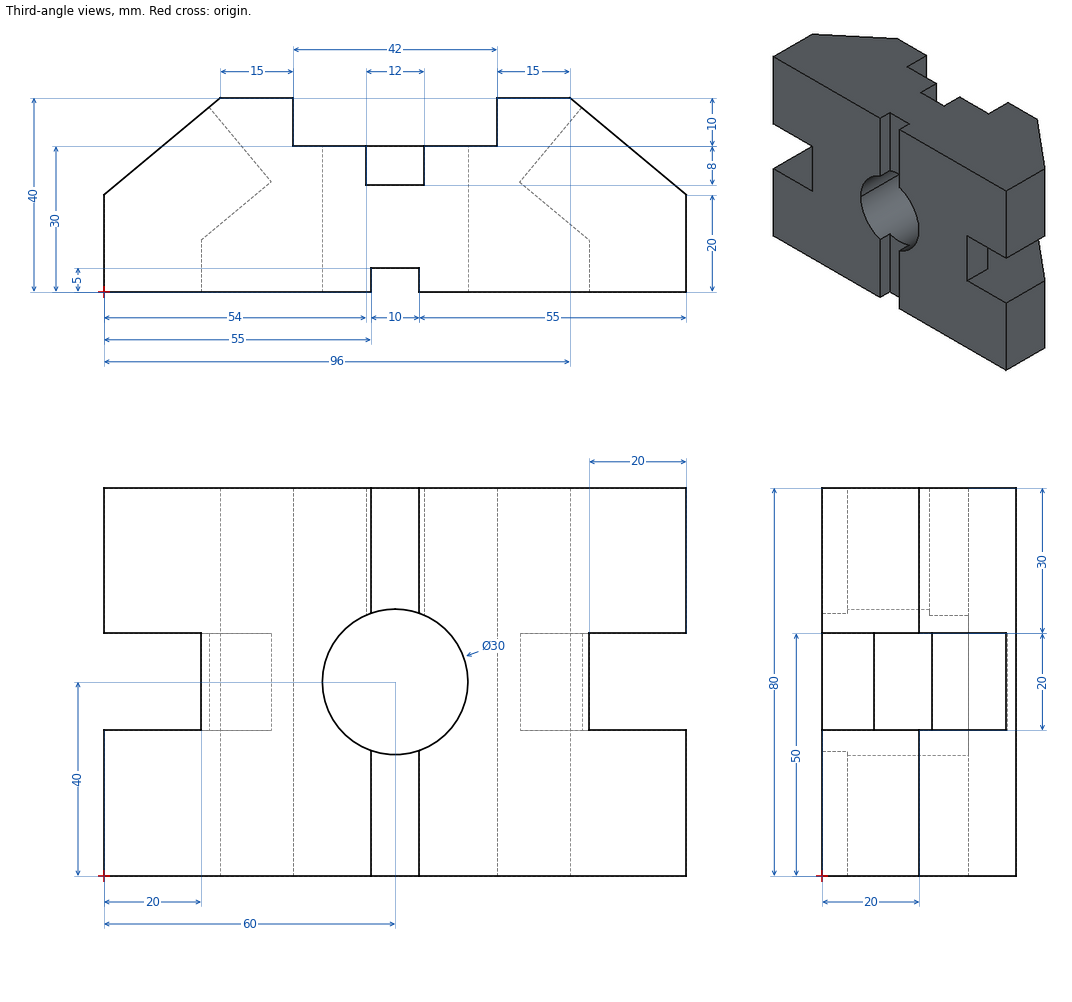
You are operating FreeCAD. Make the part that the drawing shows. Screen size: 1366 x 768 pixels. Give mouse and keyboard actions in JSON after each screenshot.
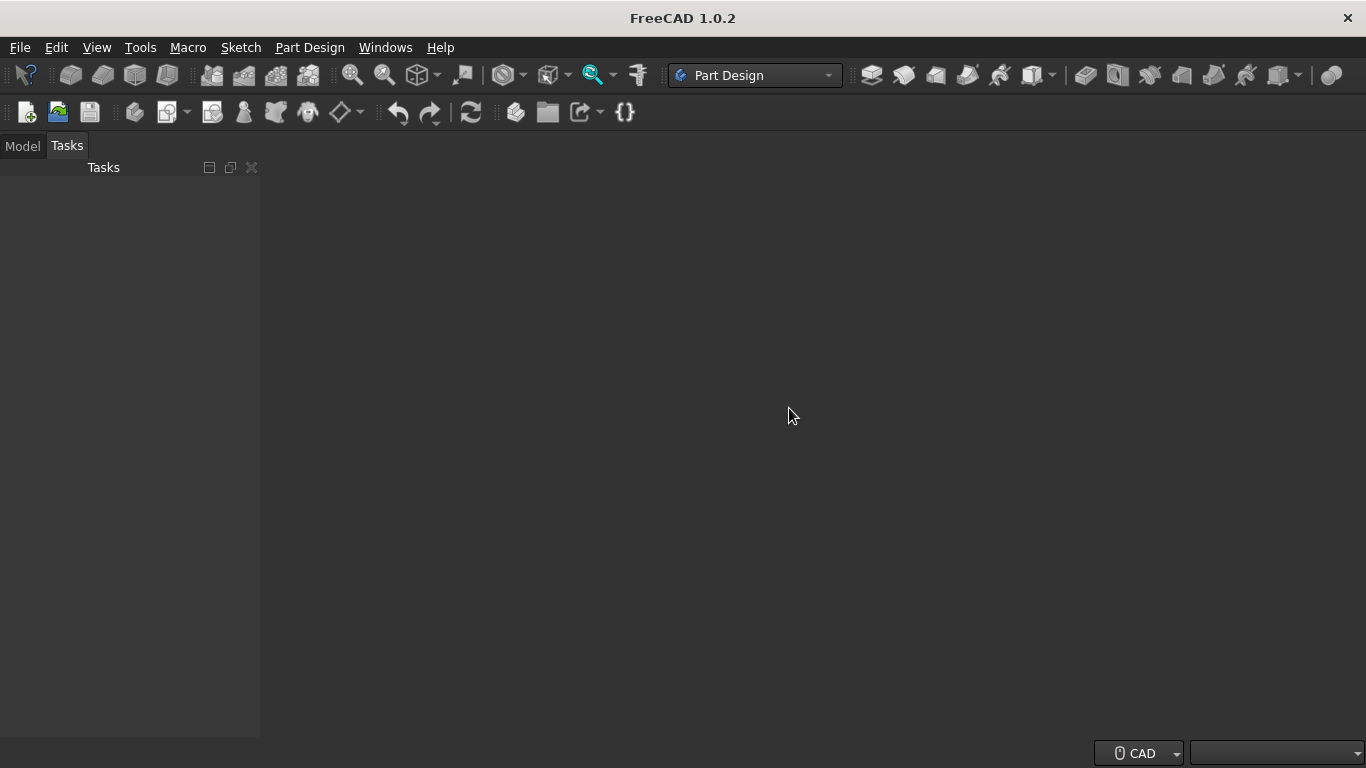
{"action": "left_click", "coordinate": [26, 112]}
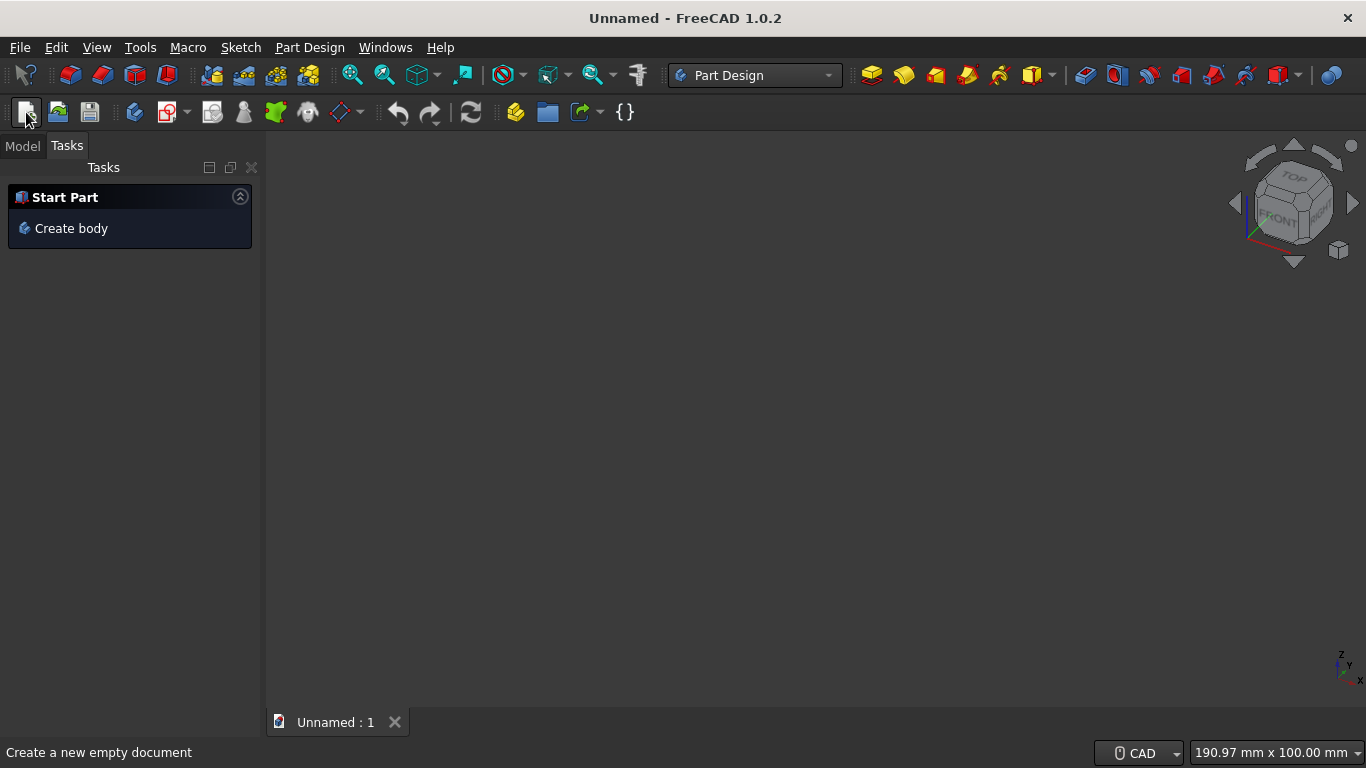
{"action": "left_click", "coordinate": [168, 112]}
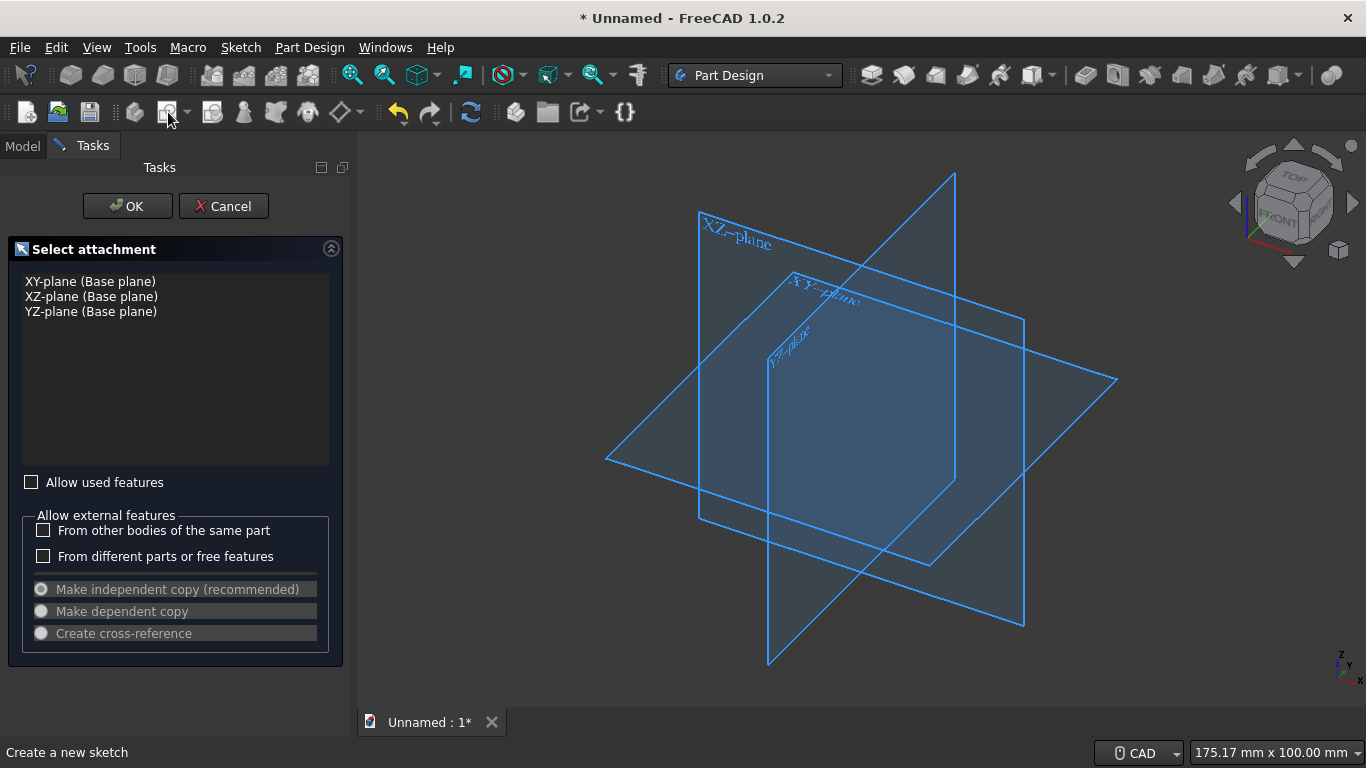
{"action": "left_click", "coordinate": [82, 282]}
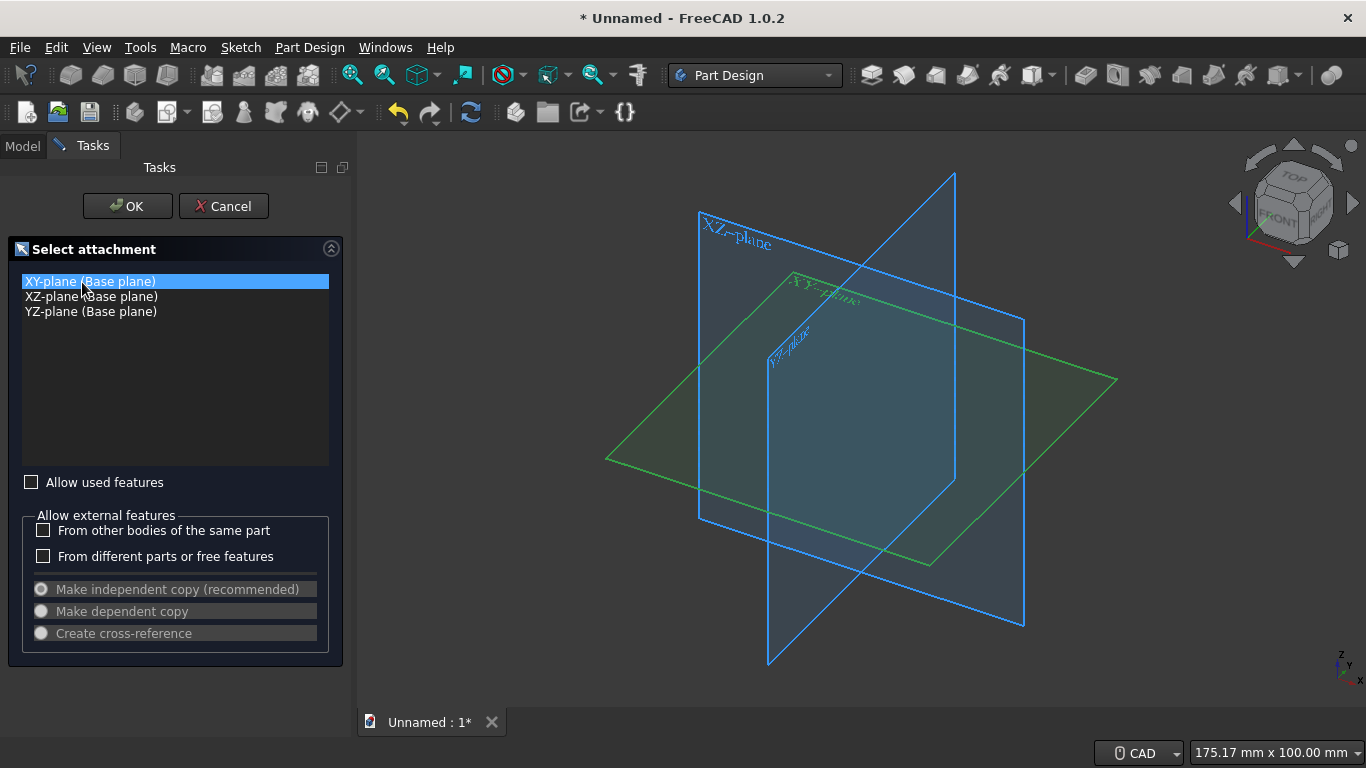
{"action": "left_click", "coordinate": [128, 206]}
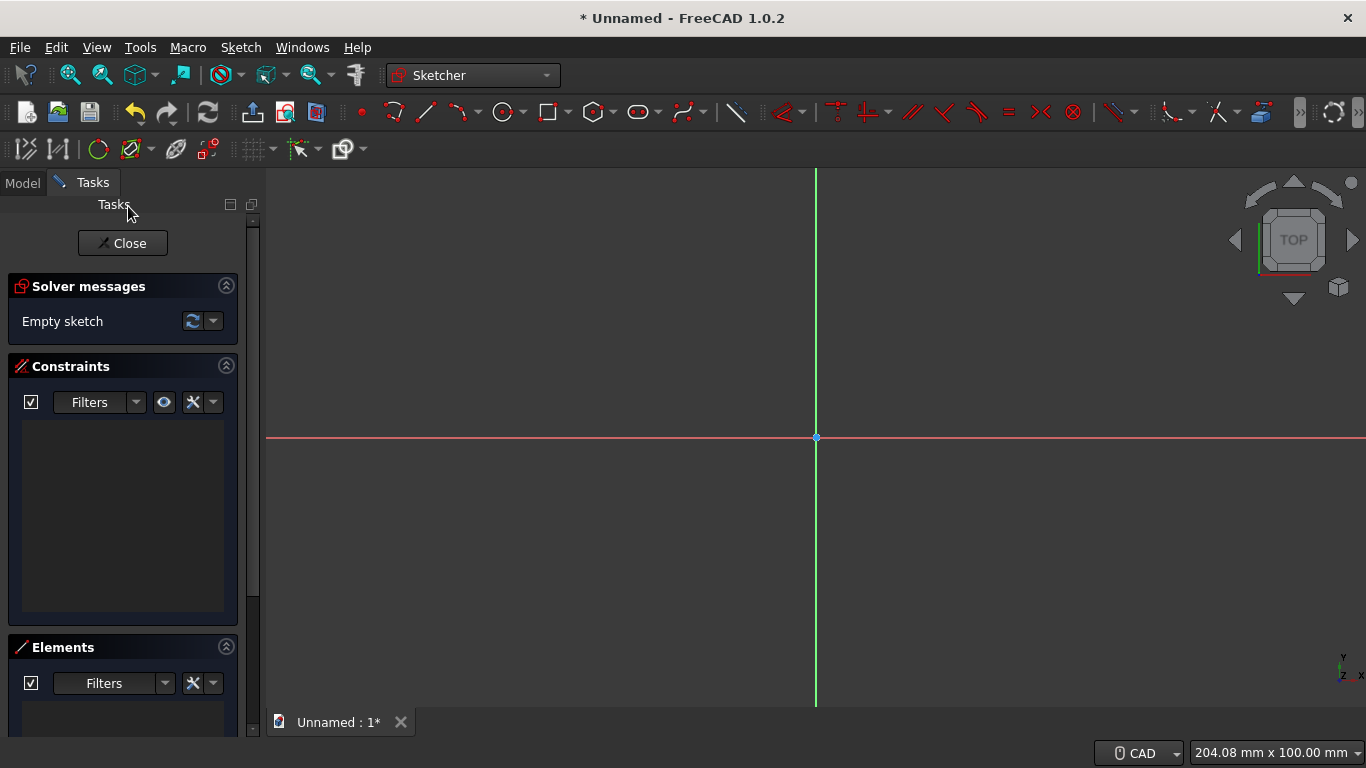
{"action": "scroll", "coordinate": [294, 657], "scroll_direction": "down", "scroll_amount": 2}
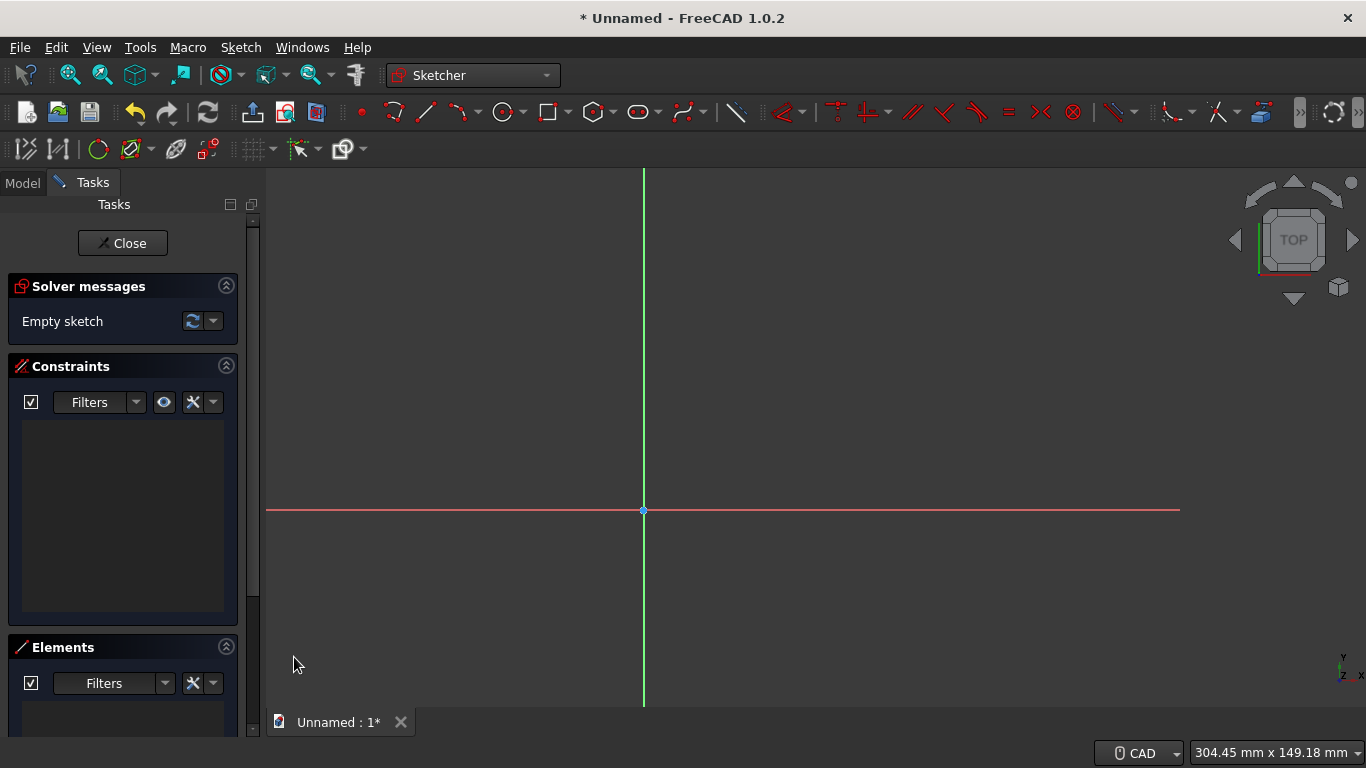
{"action": "scroll", "coordinate": [1091, 439], "scroll_direction": "up", "scroll_amount": 2}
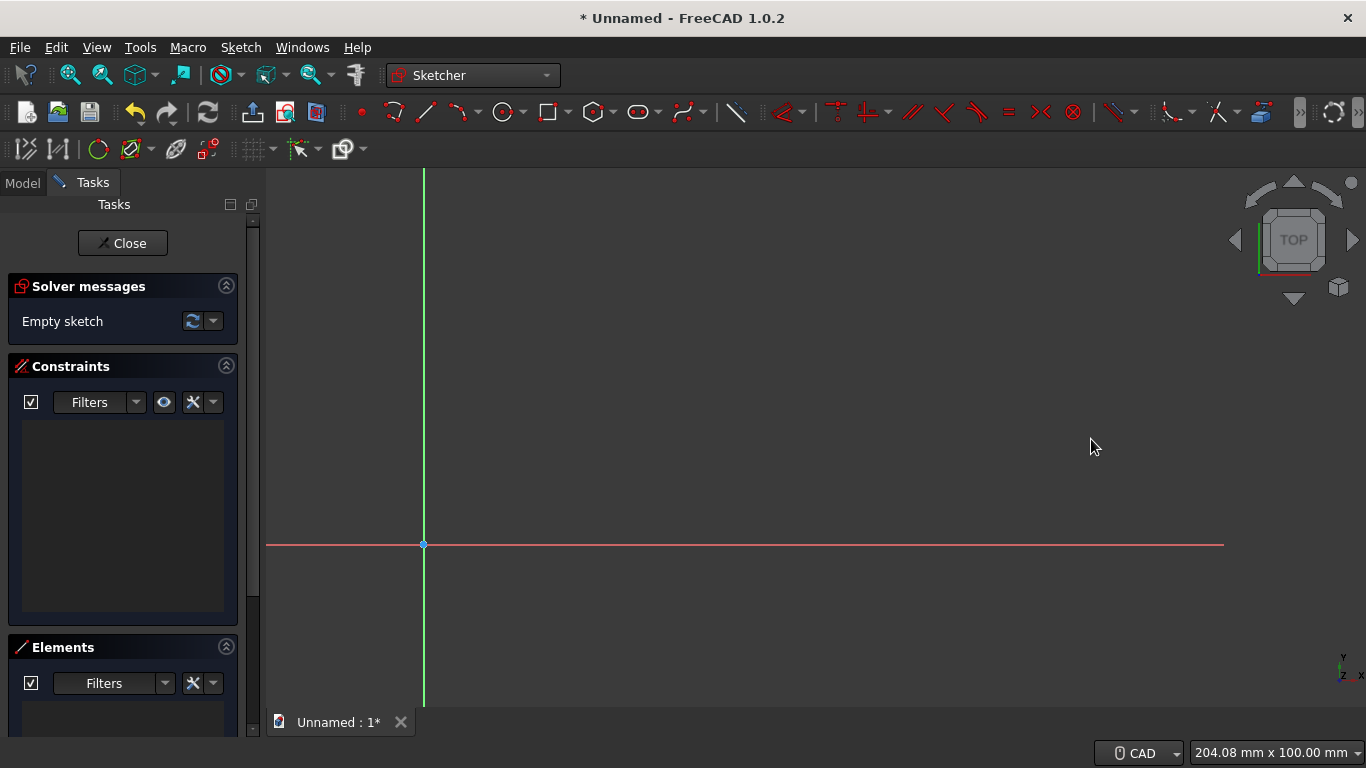
{"action": "key", "text": "g m"}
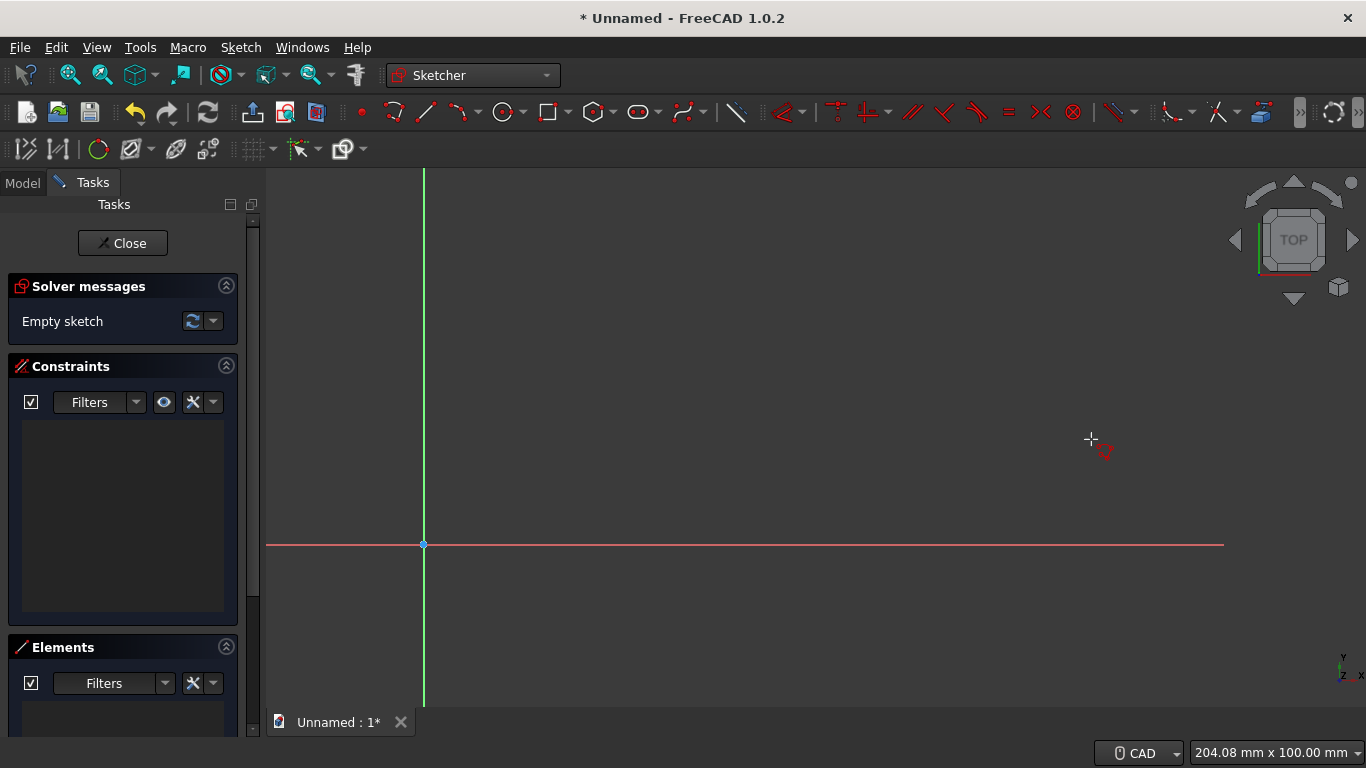
{"action": "left_click", "coordinate": [424, 545]}
{"action": "left_click", "coordinate": [720, 536]}
{"action": "left_click", "coordinate": [720, 518]}
{"action": "left_click", "coordinate": [774, 518]}
{"action": "left_click", "coordinate": [774, 545]}
{"action": "left_click", "coordinate": [1070, 536]}
{"action": "left_click", "coordinate": [1070, 437]}
{"action": "left_click", "coordinate": [941, 329]}
{"action": "left_click", "coordinate": [860, 329]}
{"action": "left_click", "coordinate": [860, 383]}
{"action": "left_click", "coordinate": [634, 383]}
{"action": "left_click", "coordinate": [634, 329]}
{"action": "left_click", "coordinate": [553, 329]}
{"action": "left_click", "coordinate": [433, 437]}
{"action": "left_click", "coordinate": [424, 545]}
{"action": "key", "text": "Escape"}
{"action": "key", "text": "Escape"}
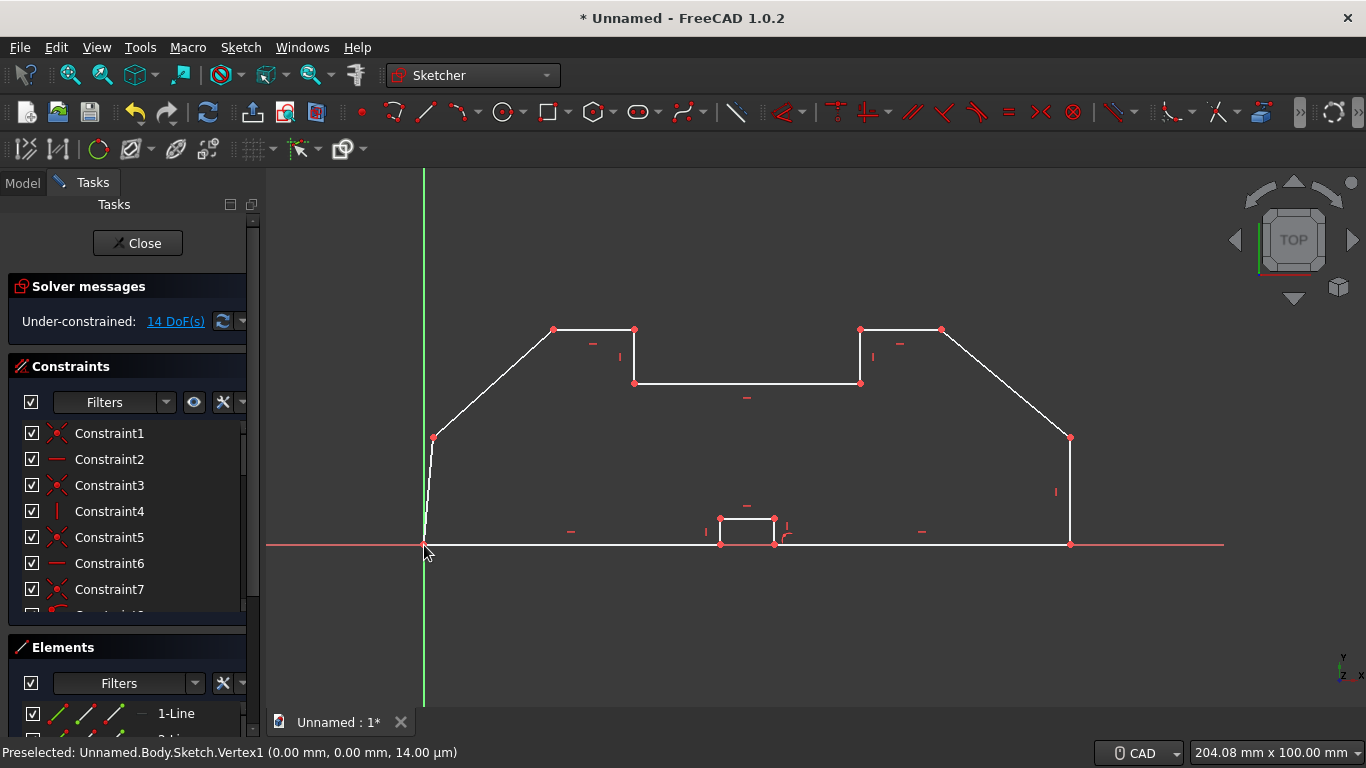
{"action": "left_click", "coordinate": [426, 513]}